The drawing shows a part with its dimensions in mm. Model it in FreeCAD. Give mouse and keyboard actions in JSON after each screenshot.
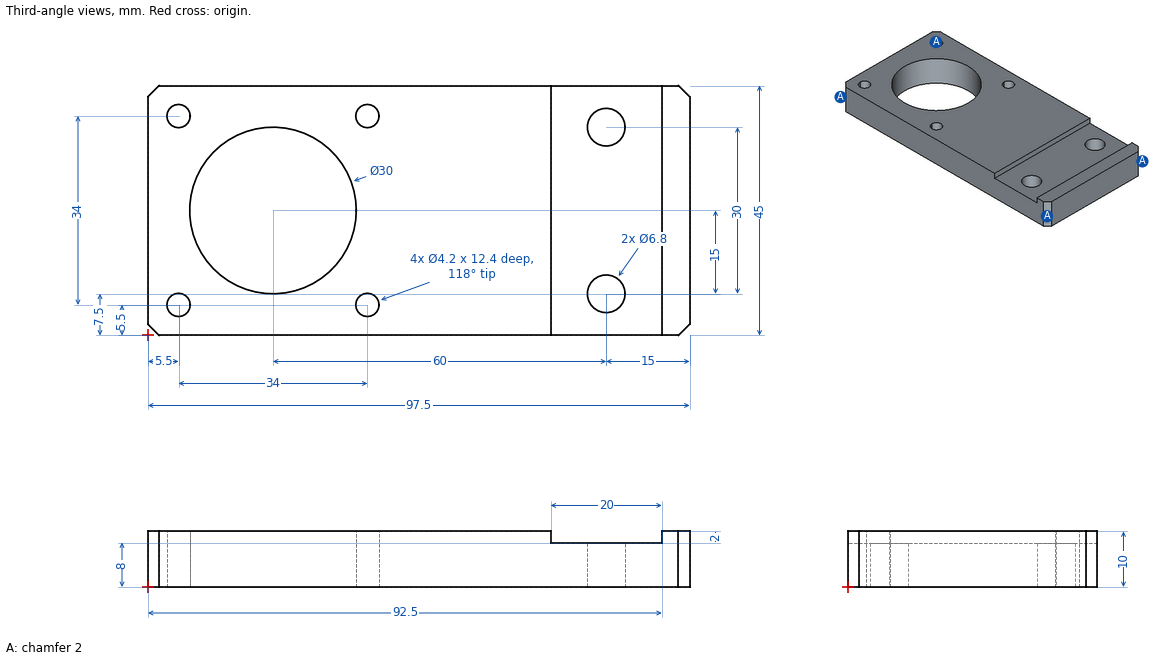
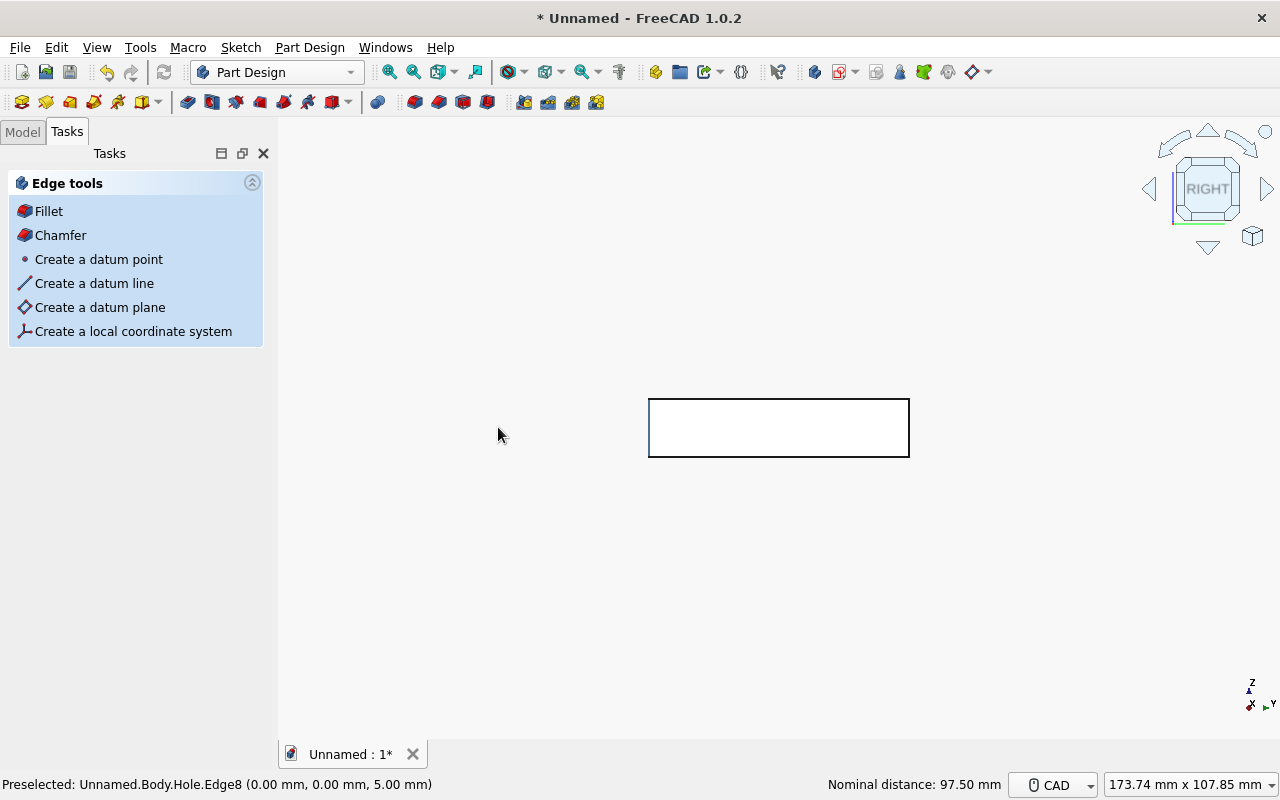
{"action": "key", "text": "v f"}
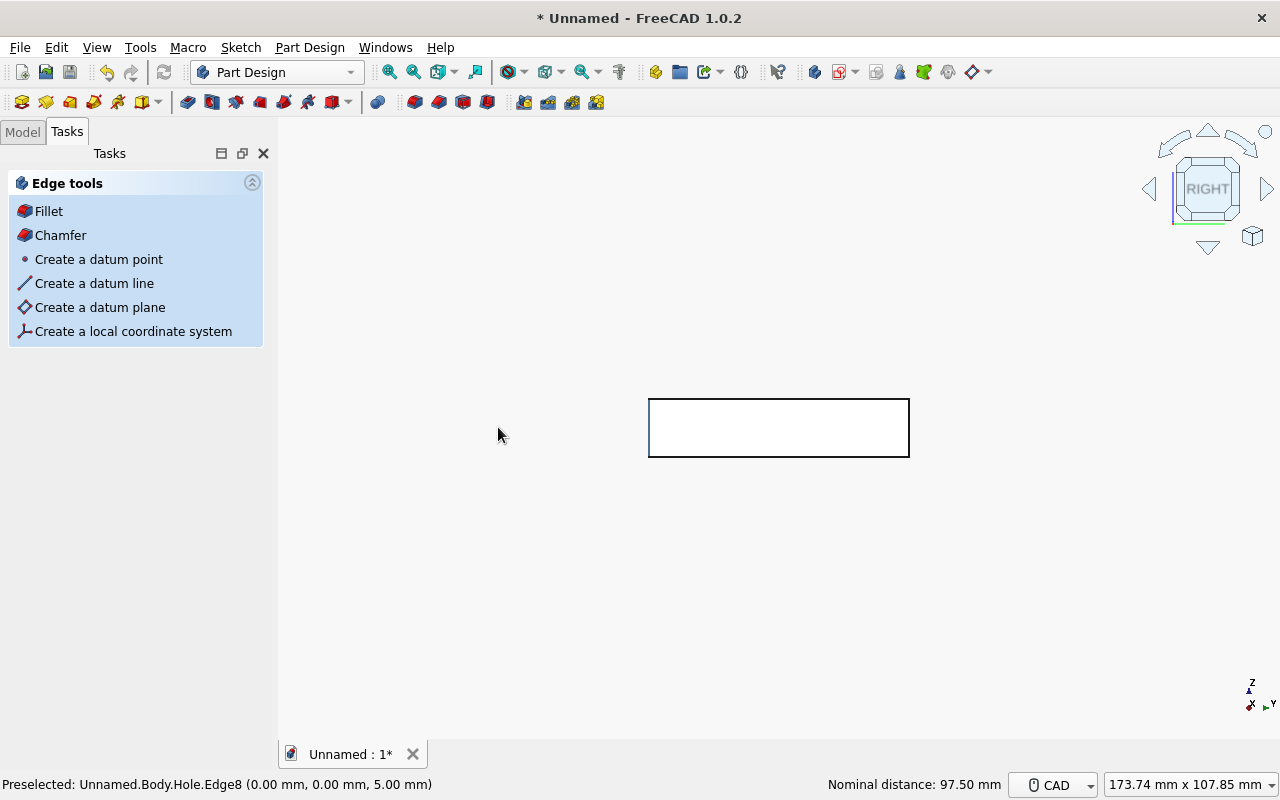
{"action": "left_click", "coordinate": [909, 427], "text": "ctrl"}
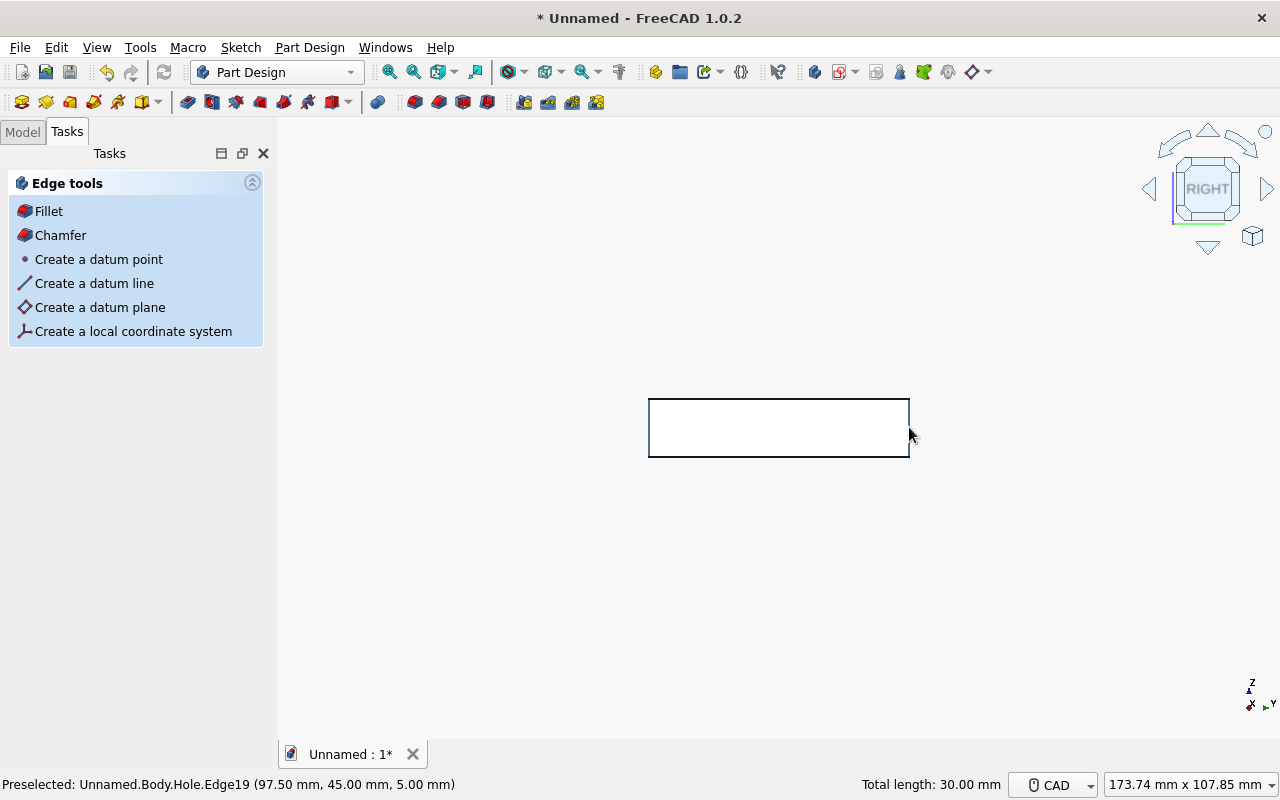
{"action": "key", "text": "5"}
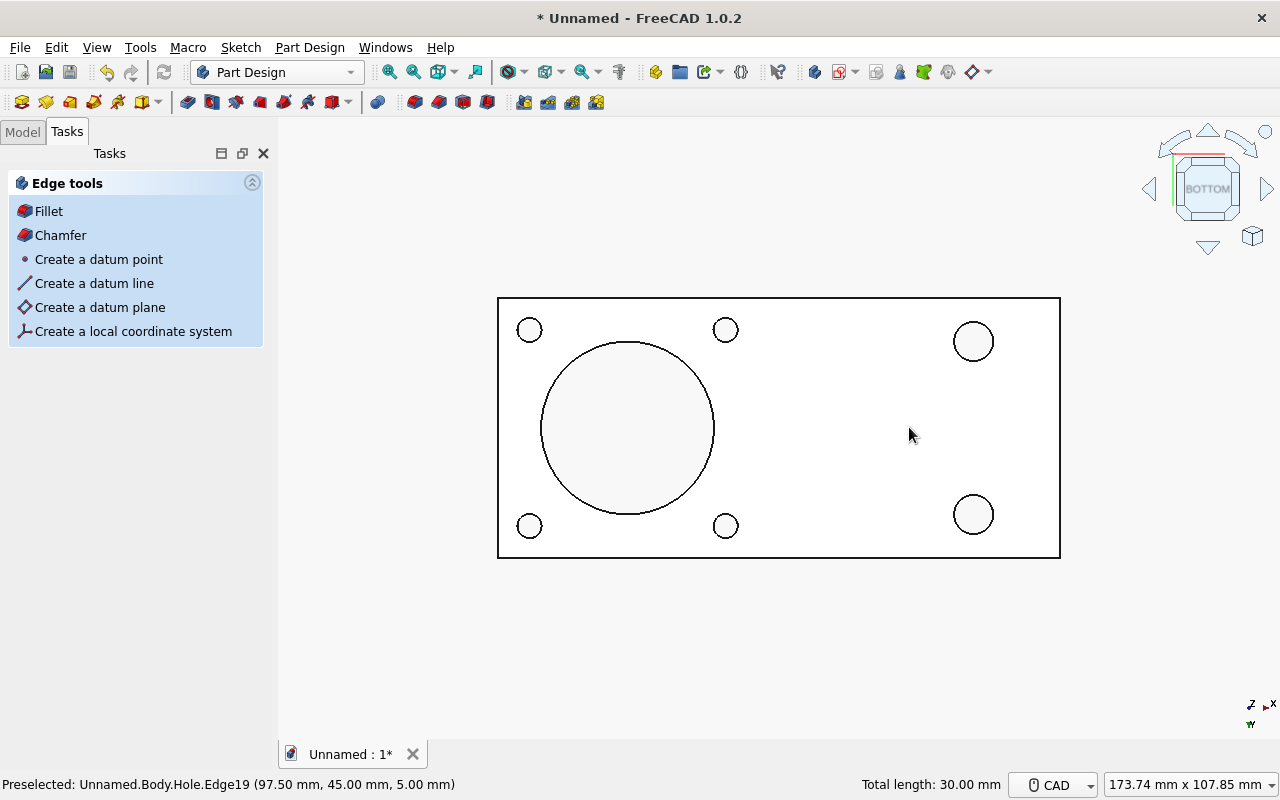
{"action": "key", "text": "4"}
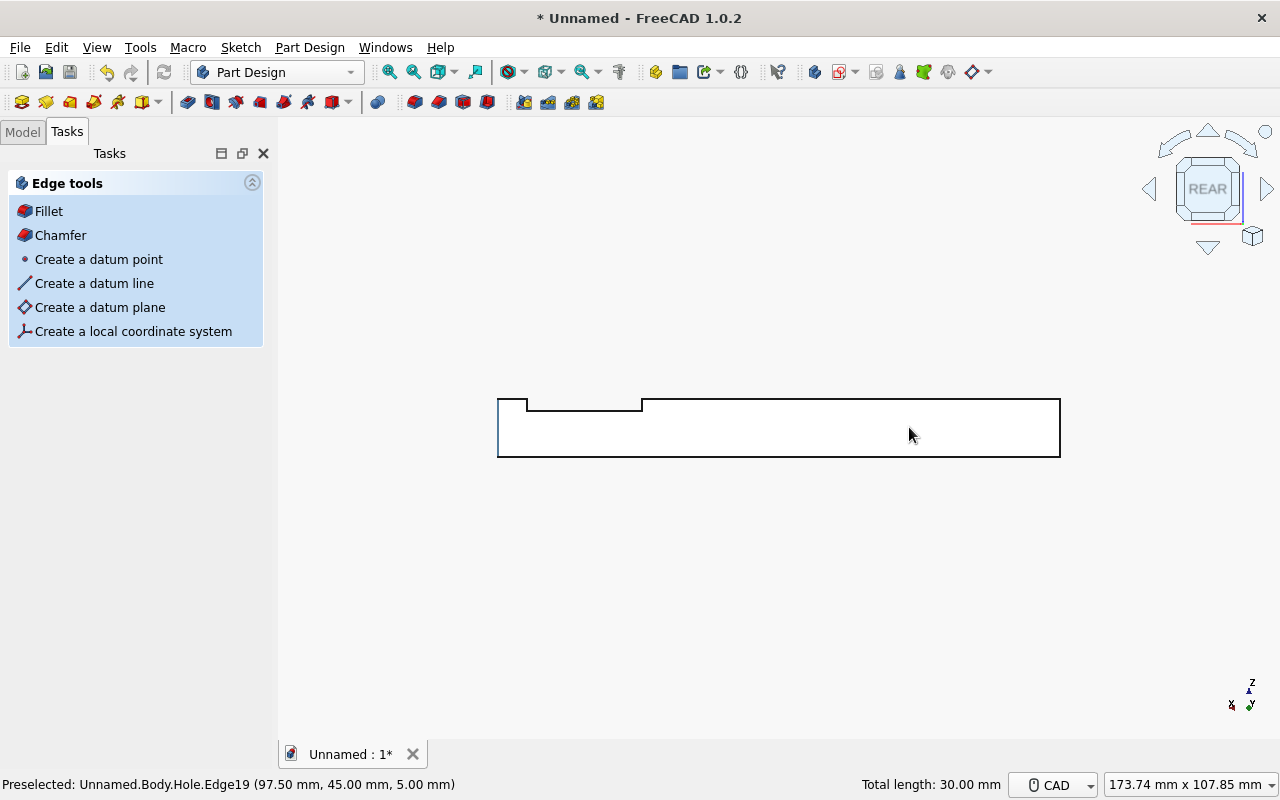
{"action": "left_click", "coordinate": [1060, 427], "text": "ctrl"}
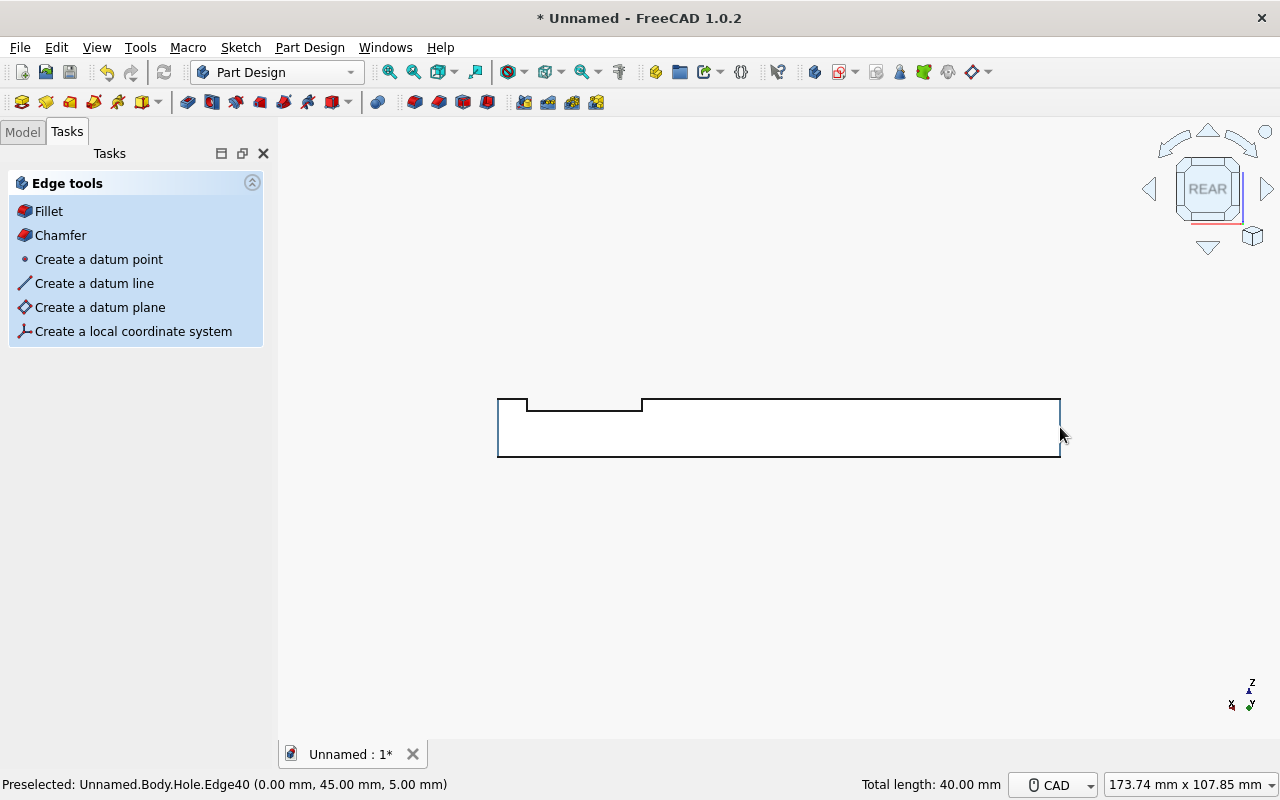
{"action": "left_click", "coordinate": [440, 102]}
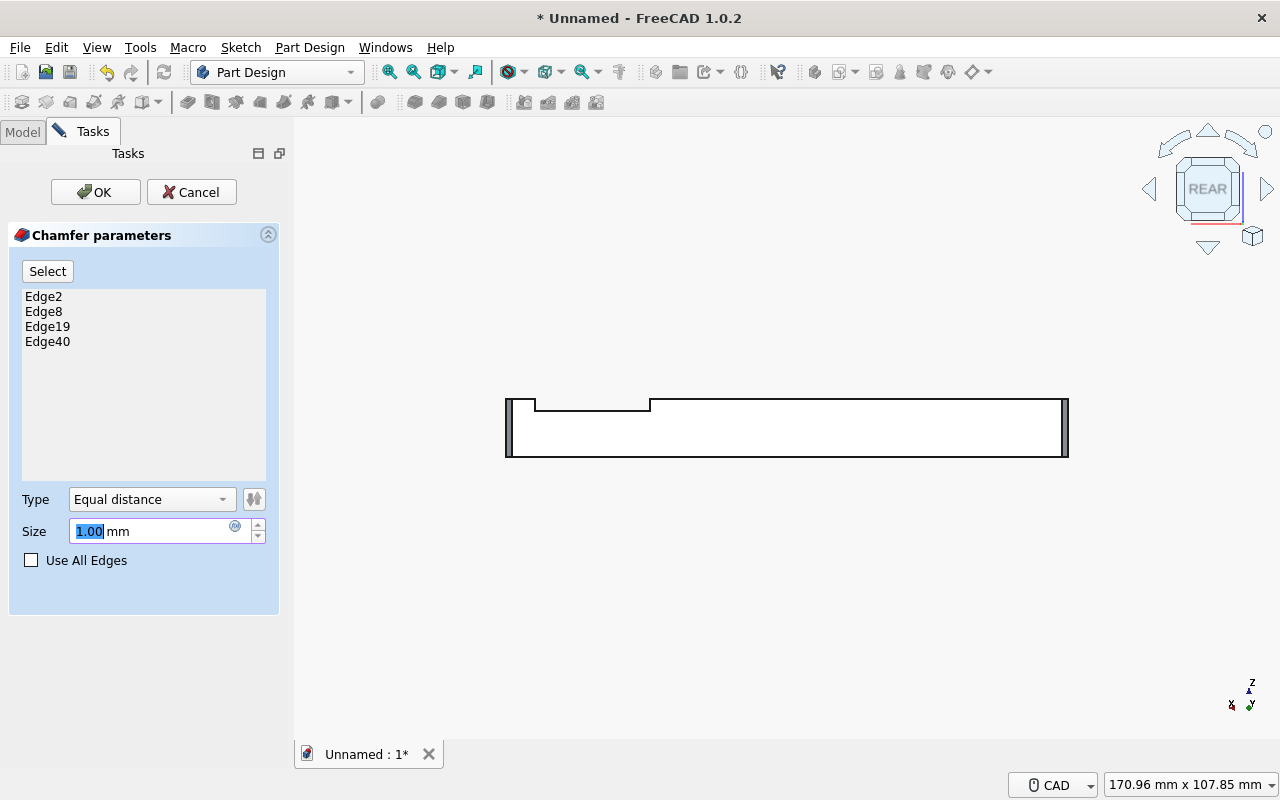
{"action": "type", "text": "2"}
{"action": "key", "text": "Tab"}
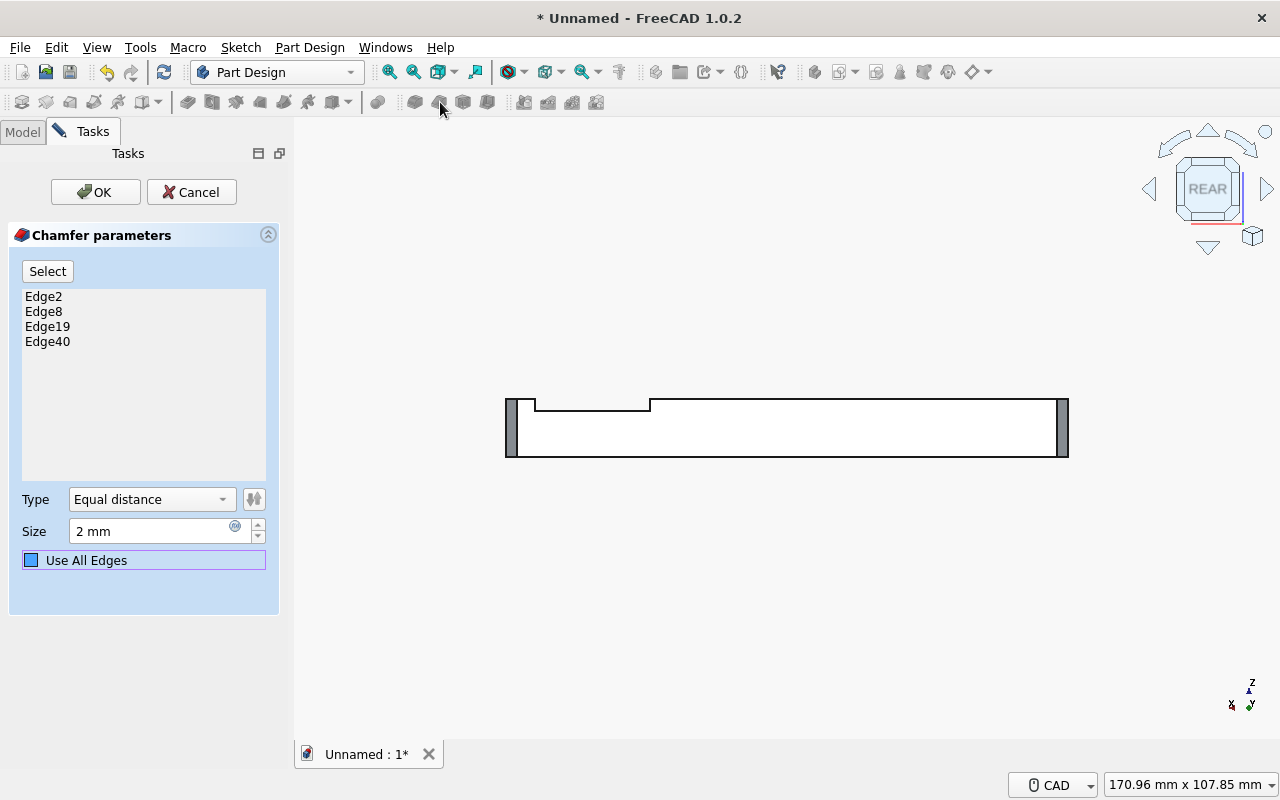
{"action": "left_click", "coordinate": [96, 192]}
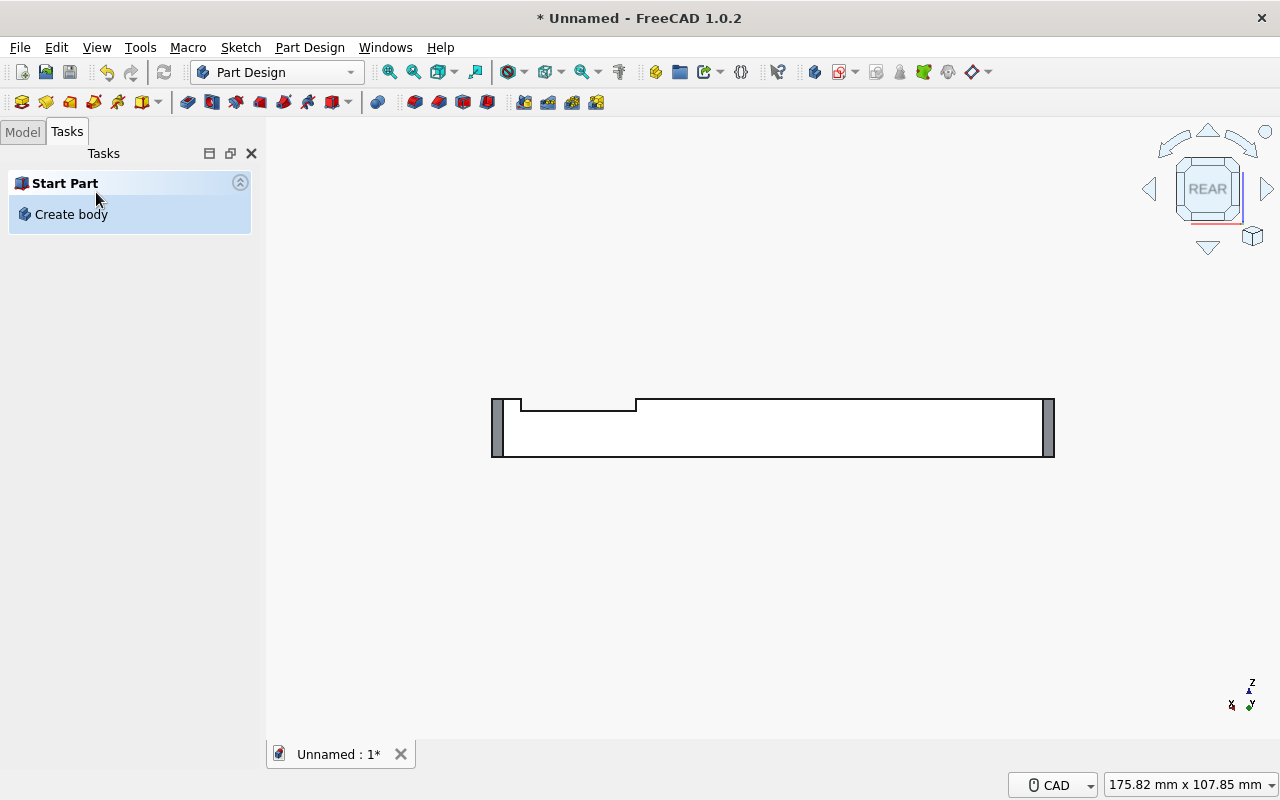
{"action": "key", "text": "0"}